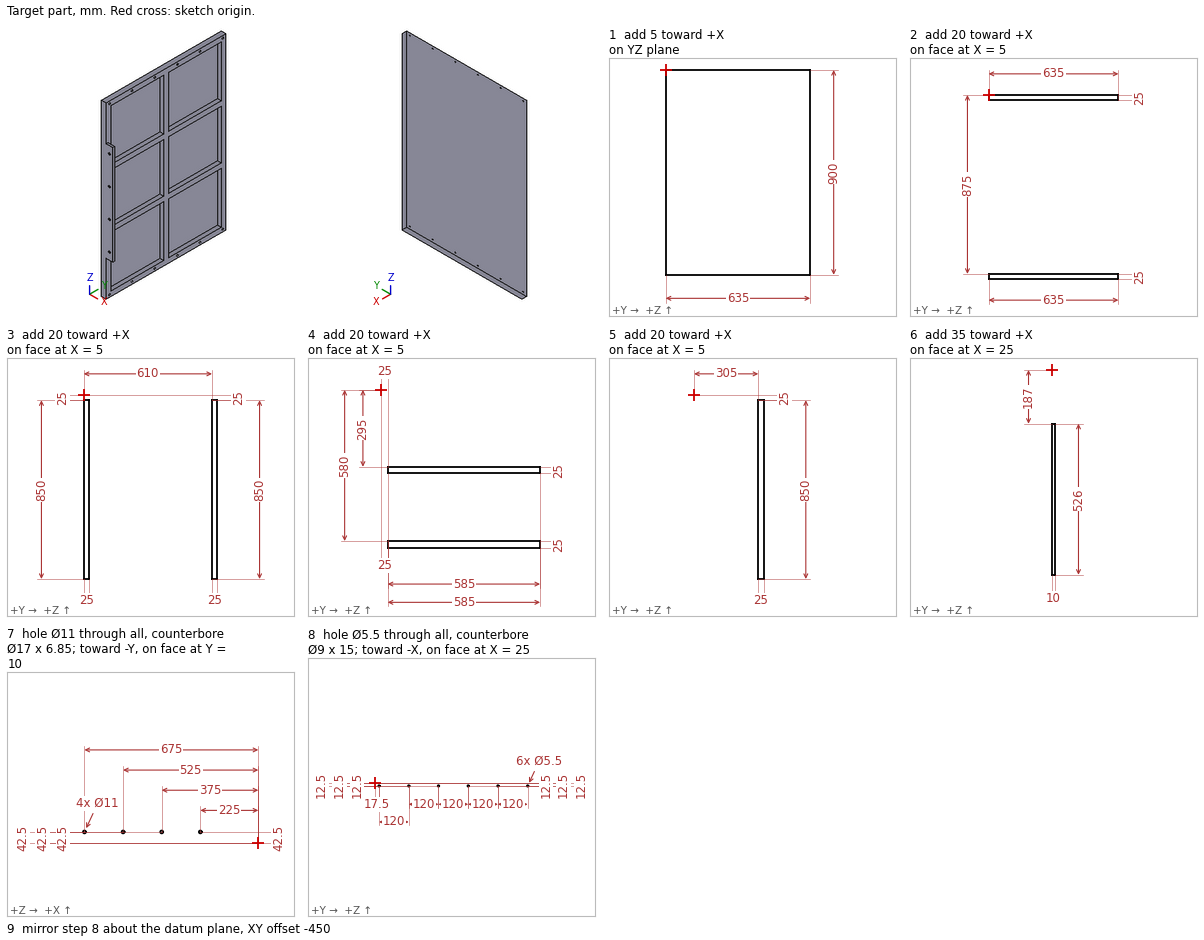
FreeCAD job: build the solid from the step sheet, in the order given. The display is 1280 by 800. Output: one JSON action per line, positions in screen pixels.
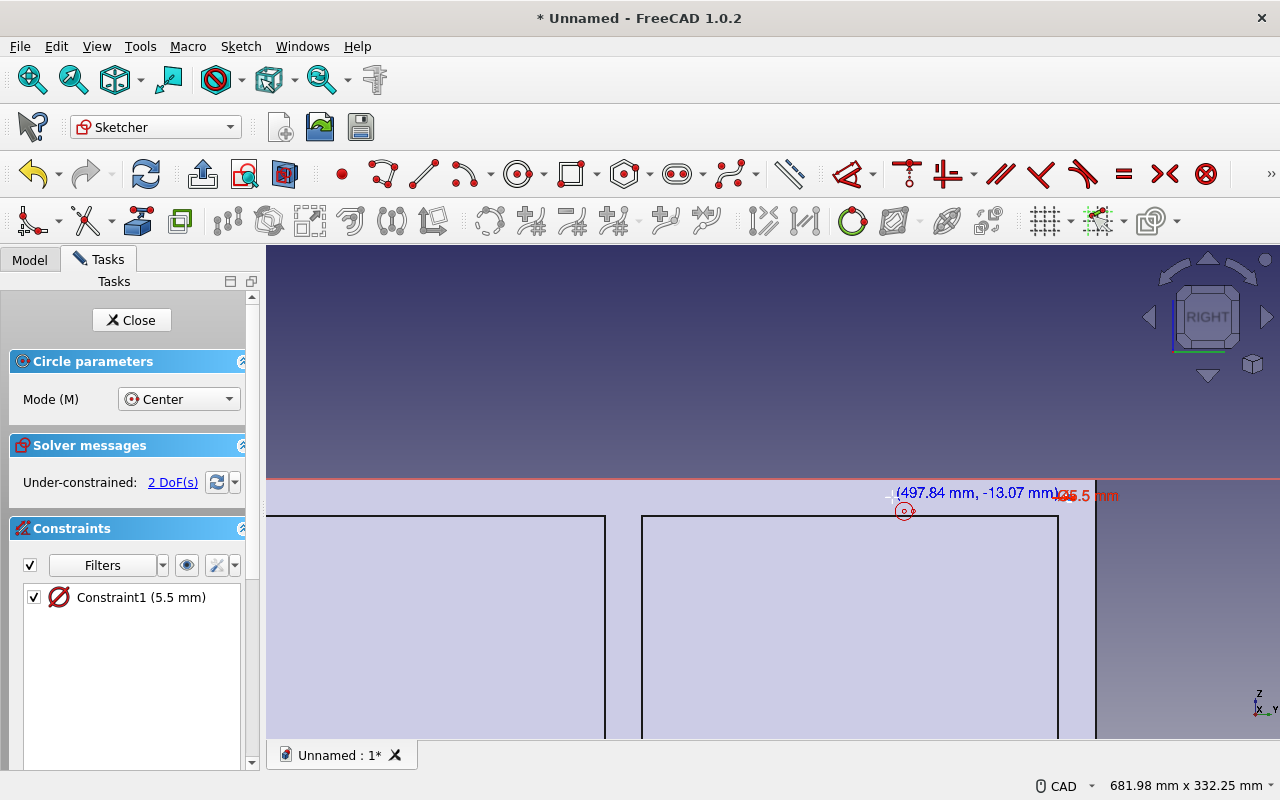
{"action": "left_click", "coordinate": [891, 497]}
{"action": "mouse_move", "coordinate": [894, 494]}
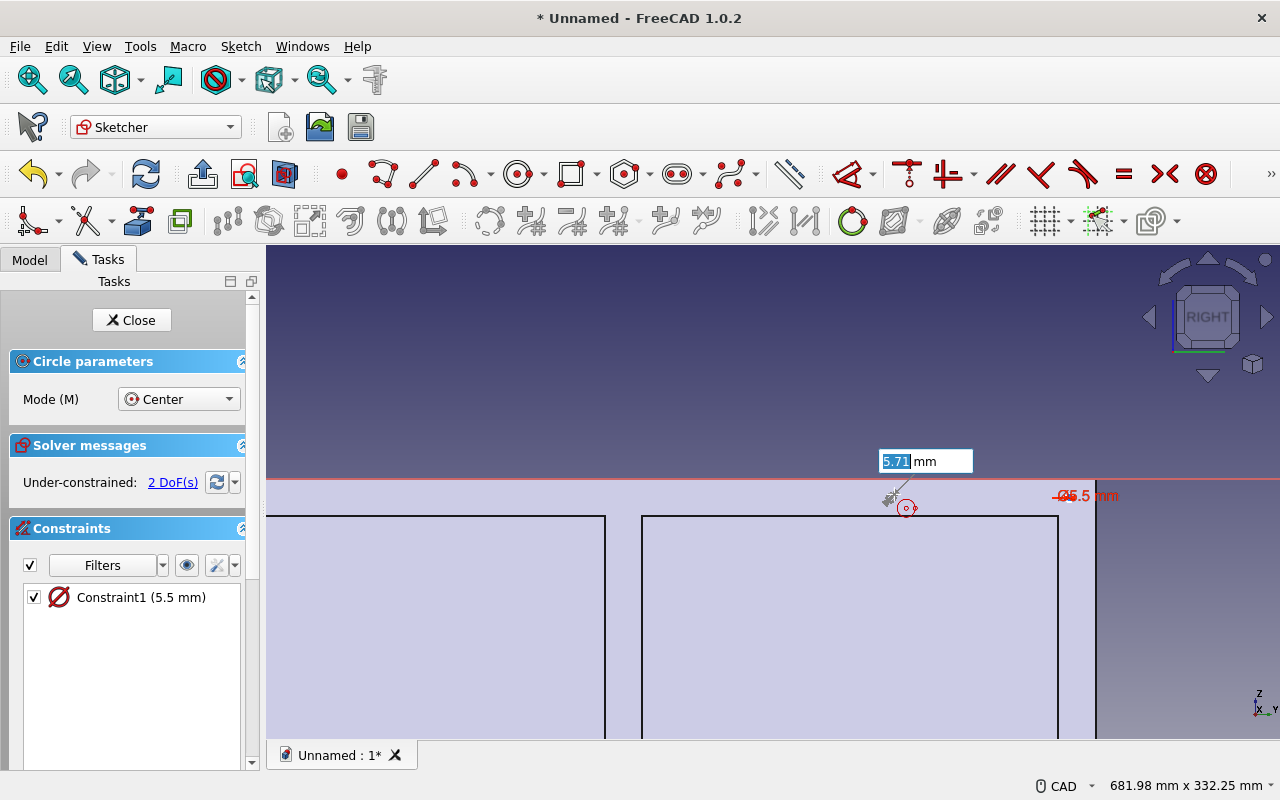
{"action": "type", "text": "5.5"}
{"action": "key", "text": "Return"}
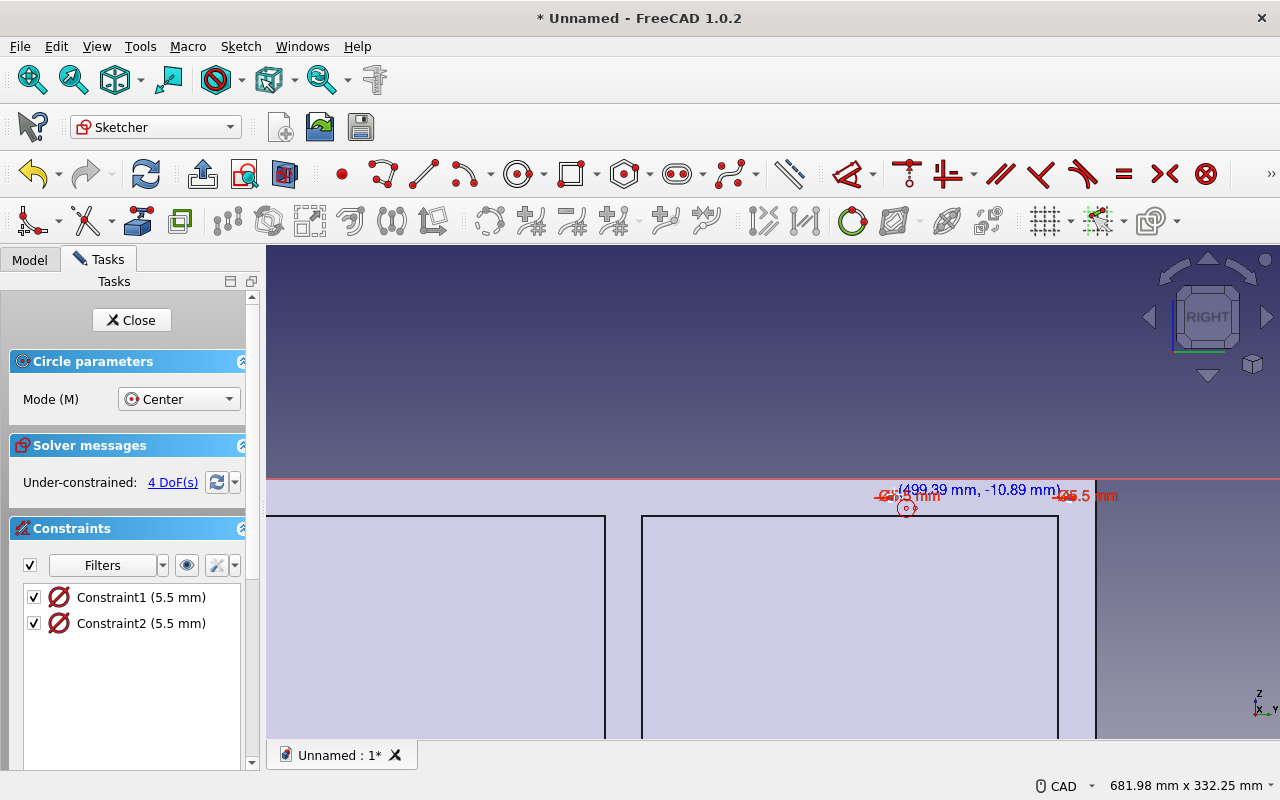
{"action": "scroll", "coordinate": [713, 497], "scroll_direction": "up", "scroll_amount": 9}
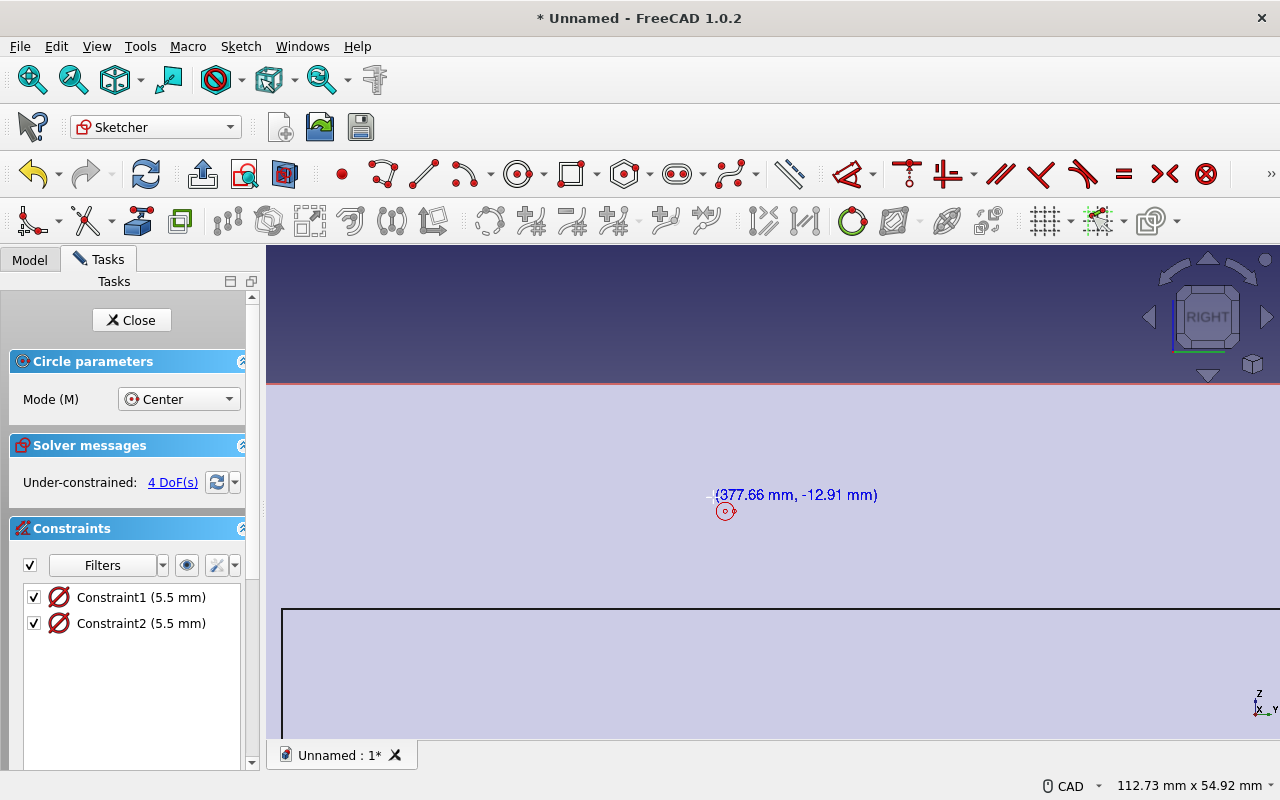
{"action": "scroll", "coordinate": [779, 497], "scroll_direction": "down", "scroll_amount": 11}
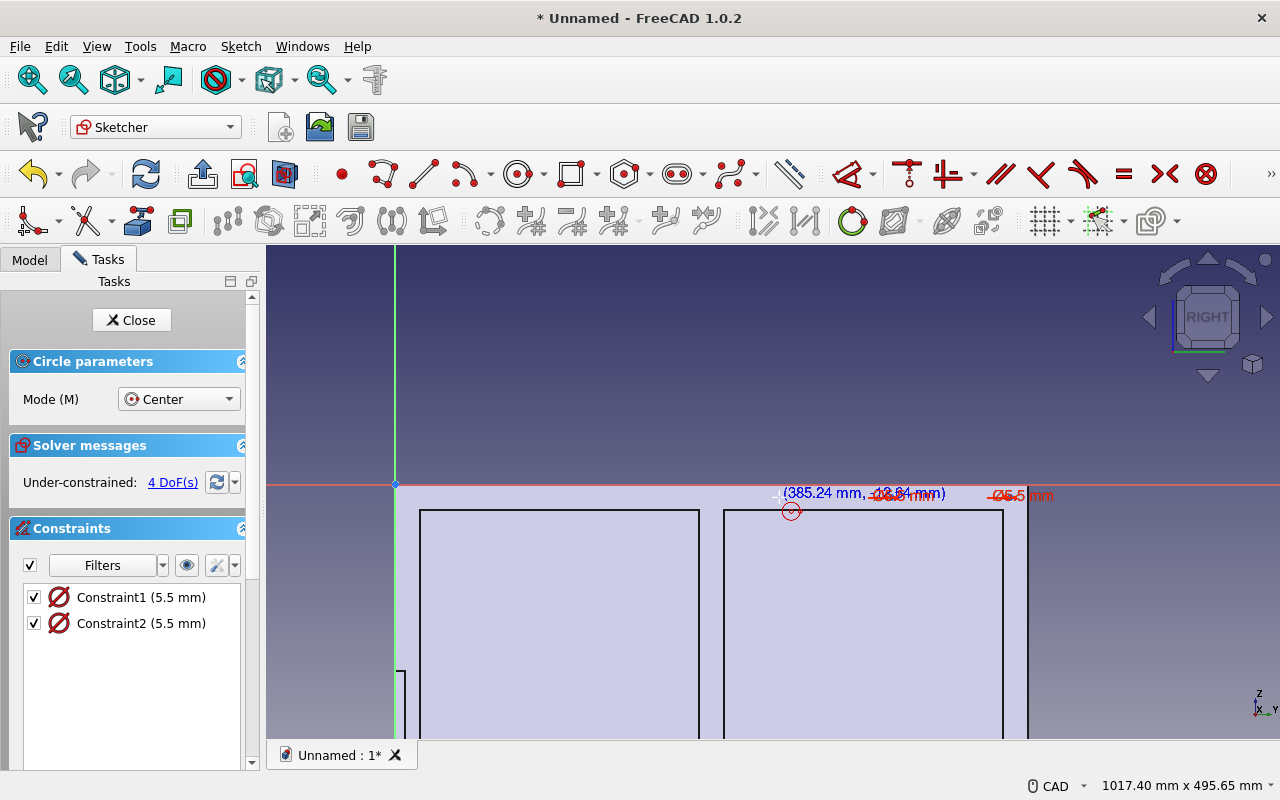
{"action": "scroll", "coordinate": [772, 497], "scroll_direction": "up", "scroll_amount": 2}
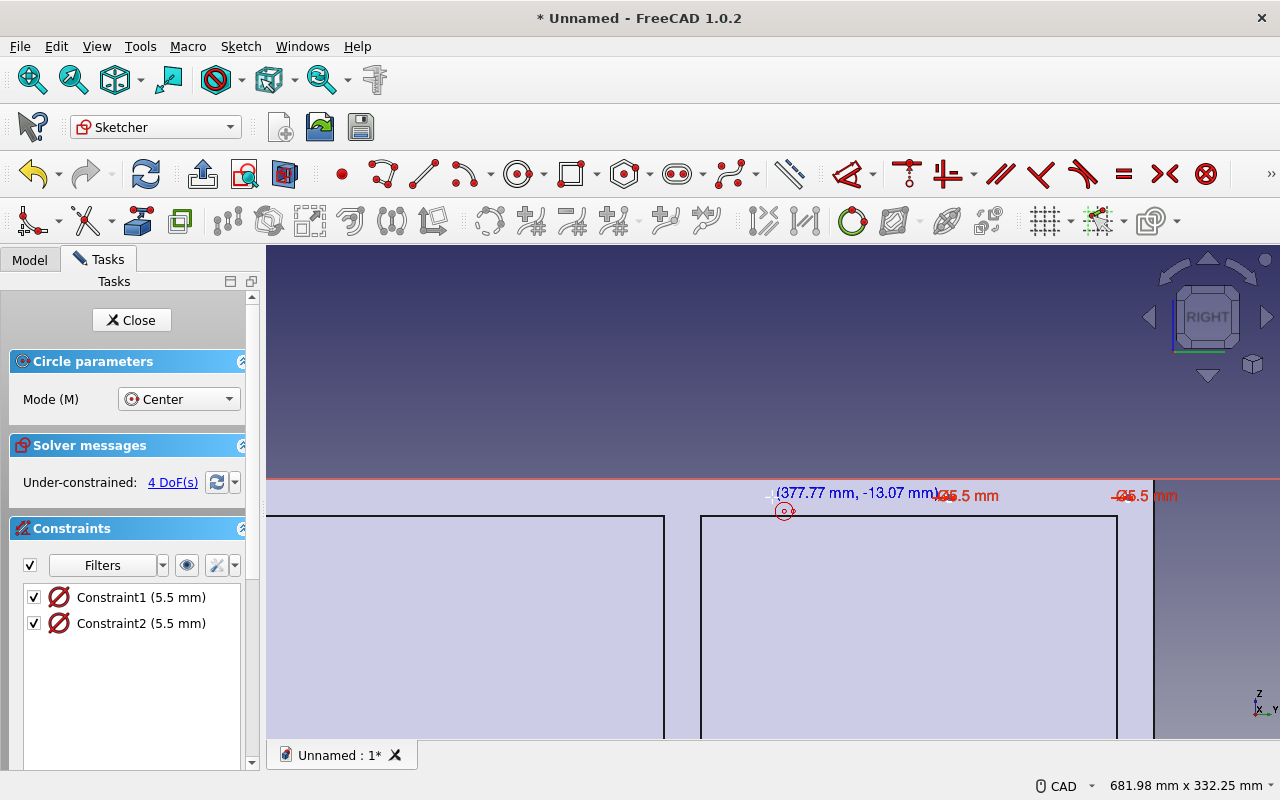
{"action": "left_click", "coordinate": [771, 497]}
{"action": "mouse_move", "coordinate": [774, 494]}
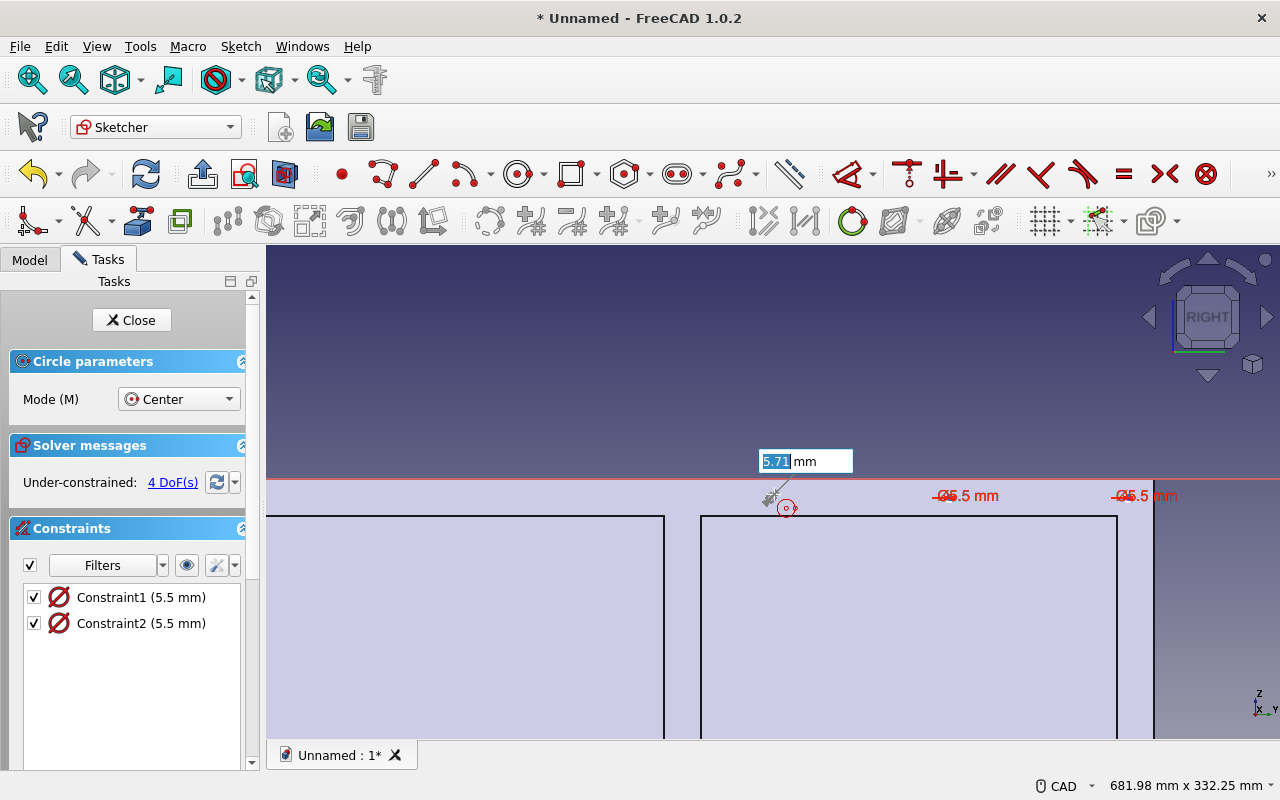
{"action": "type", "text": "5.5"}
{"action": "key", "text": "Return"}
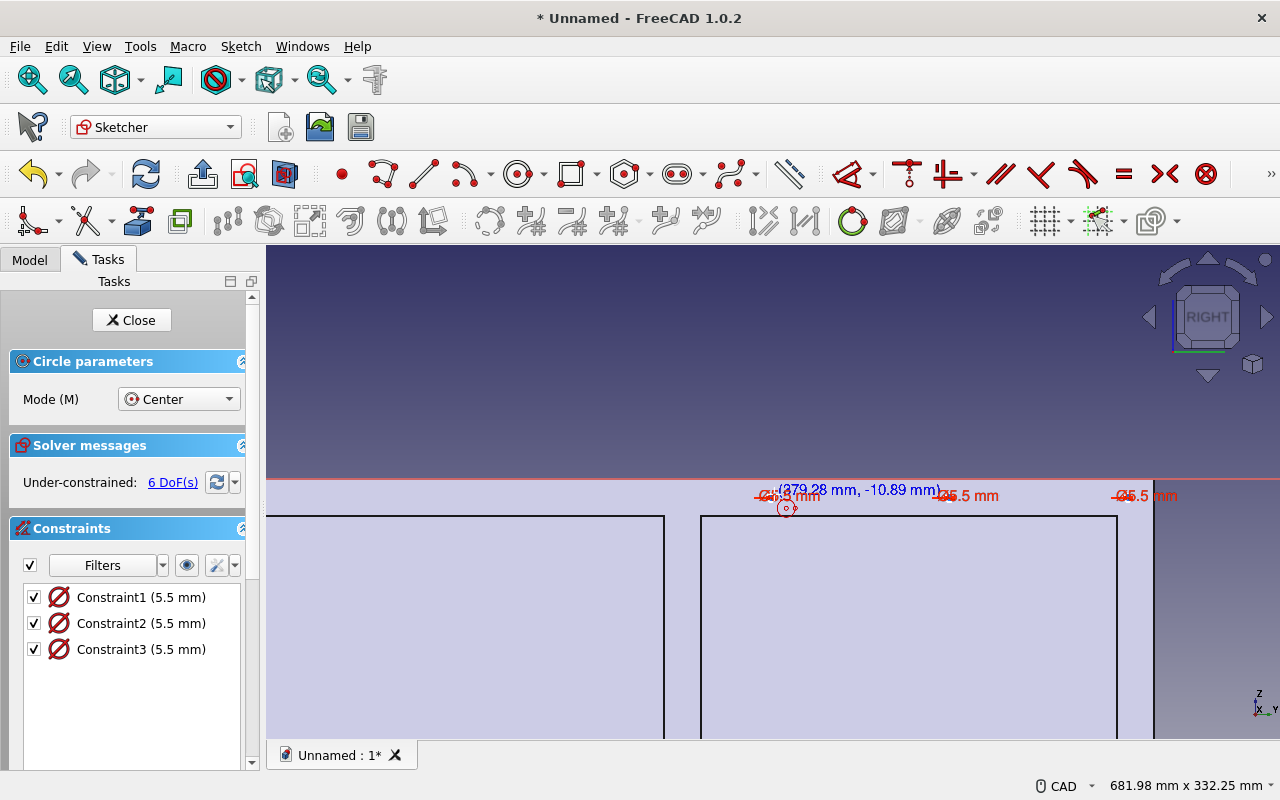
{"action": "scroll", "coordinate": [593, 497], "scroll_direction": "up", "scroll_amount": 9}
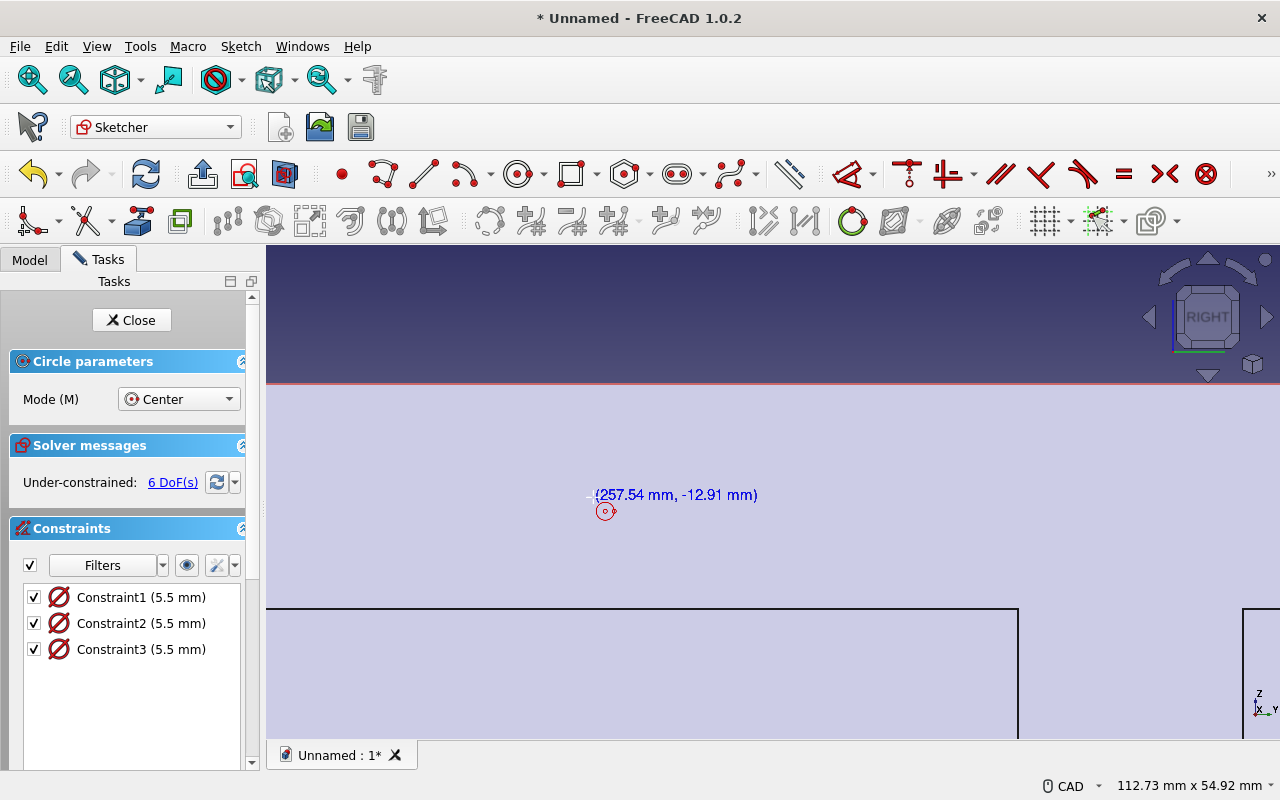
{"action": "scroll", "coordinate": [660, 497], "scroll_direction": "down", "scroll_amount": 11}